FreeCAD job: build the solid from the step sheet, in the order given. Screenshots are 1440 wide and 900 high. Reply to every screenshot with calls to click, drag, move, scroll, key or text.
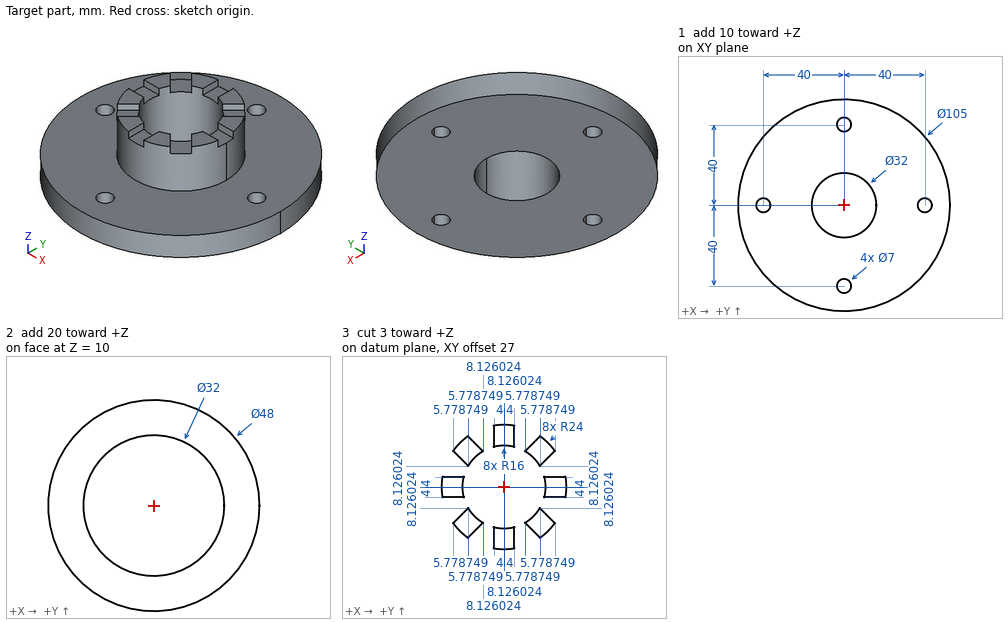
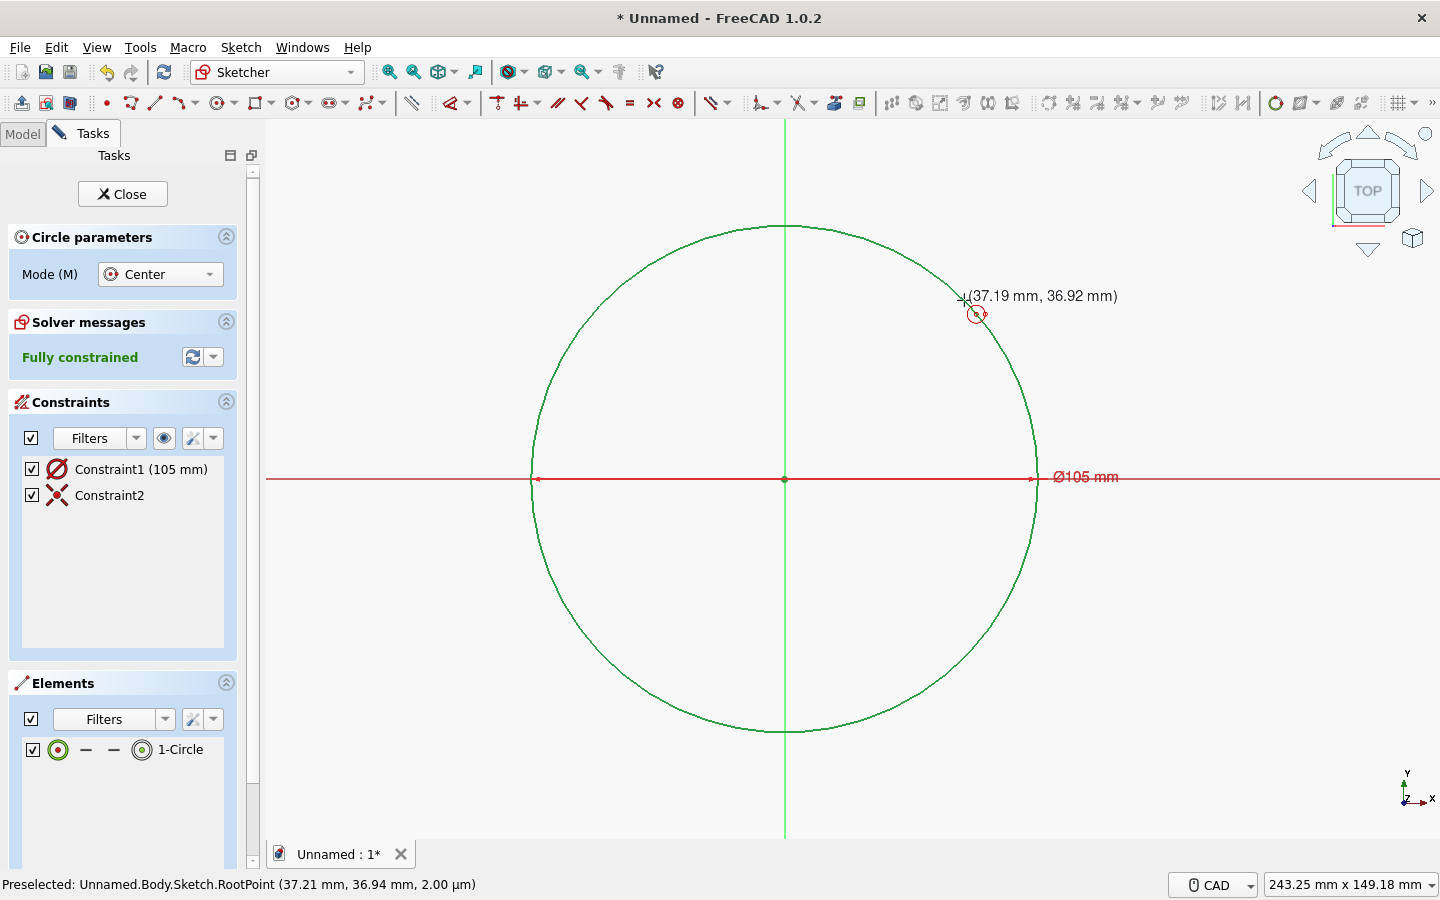
scroll(785, 672, up, 2)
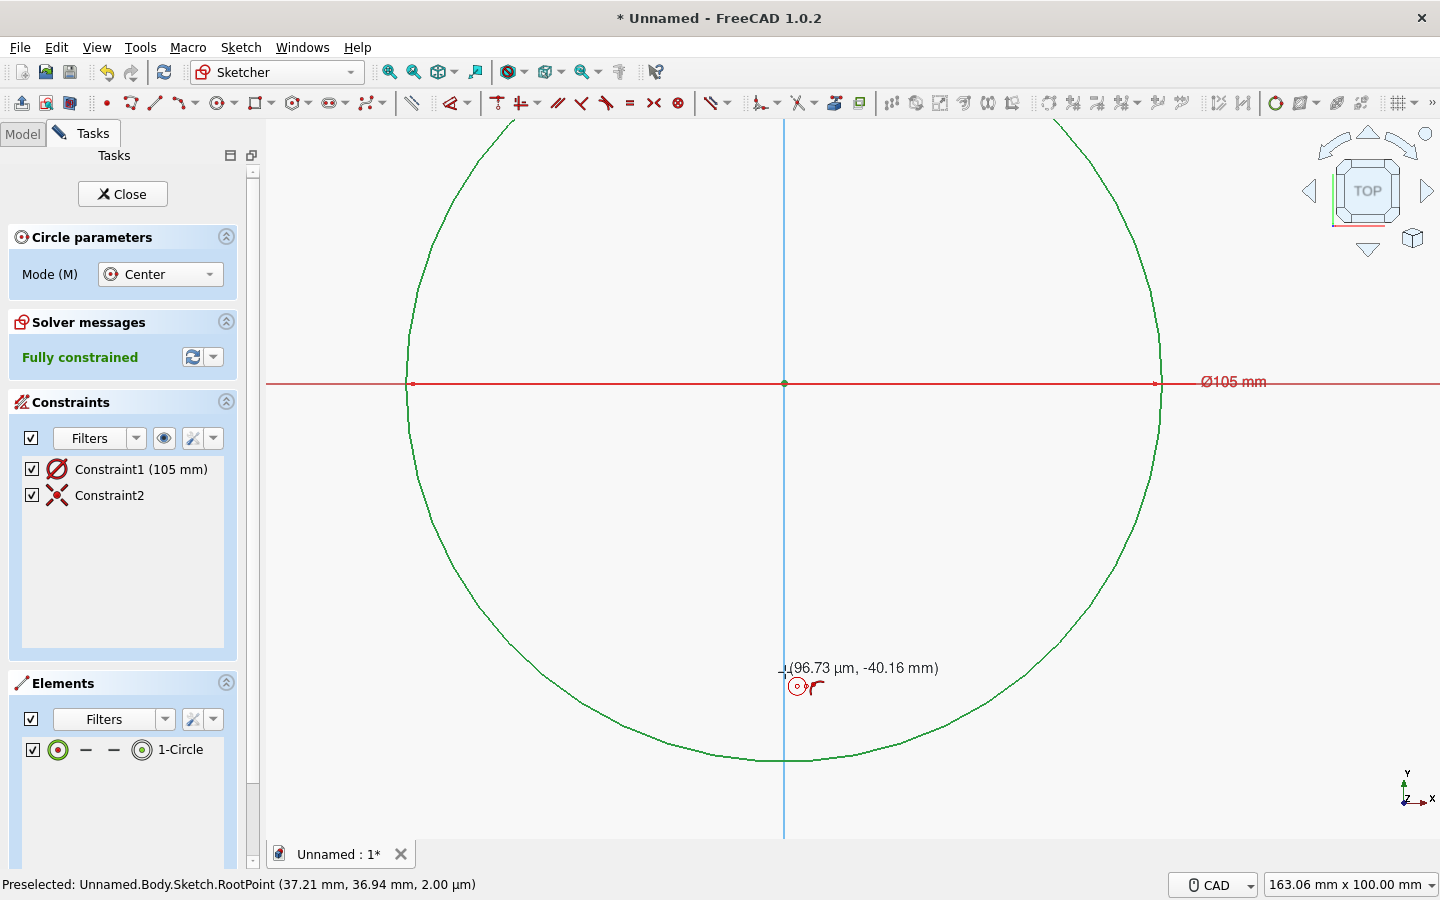
click(784, 672)
move(802, 654)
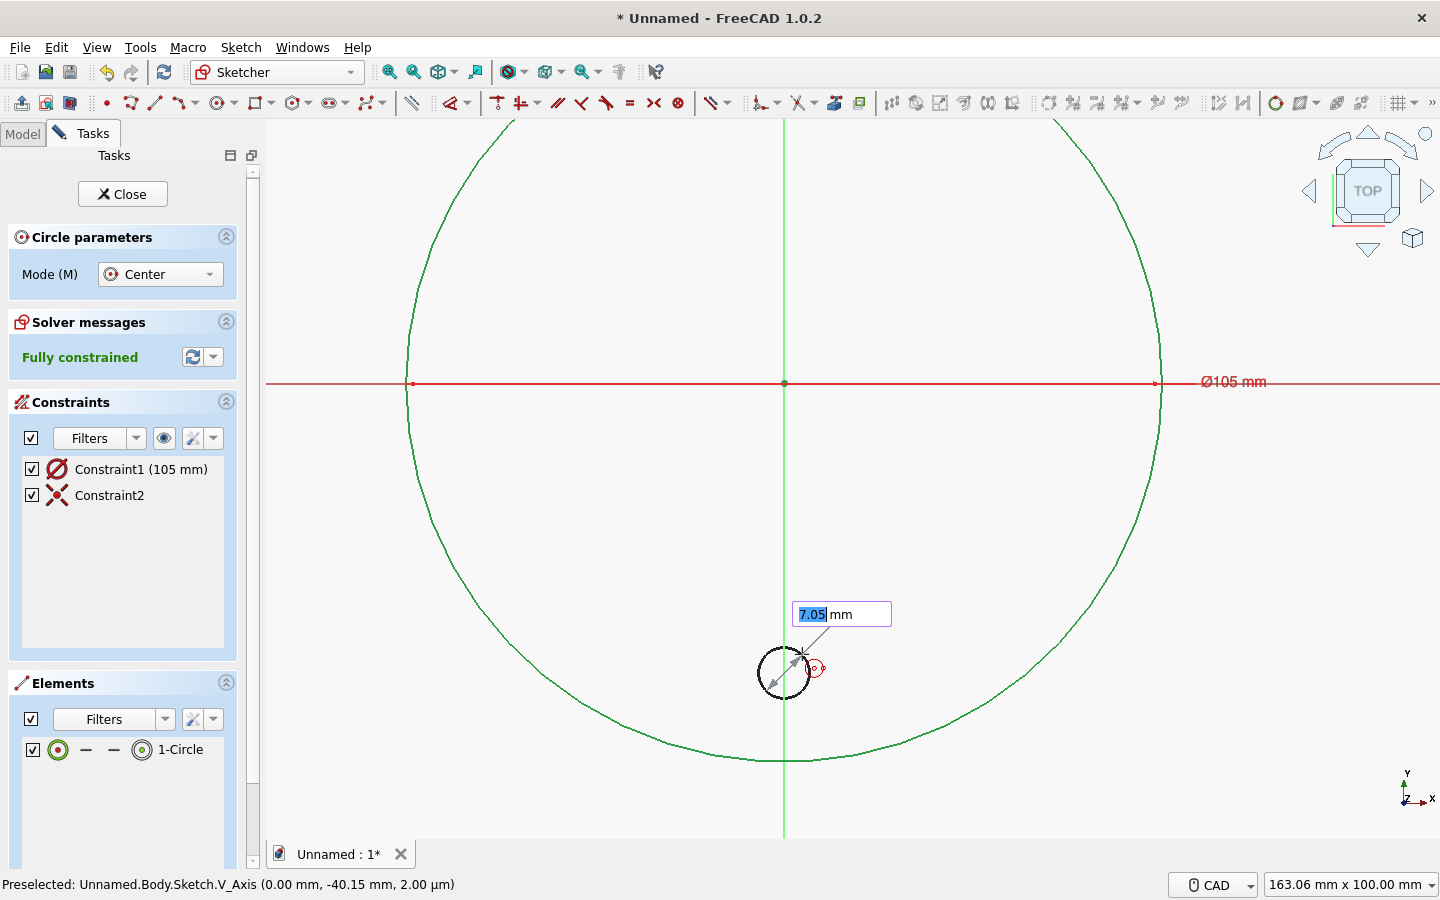
text(7)
key(Return)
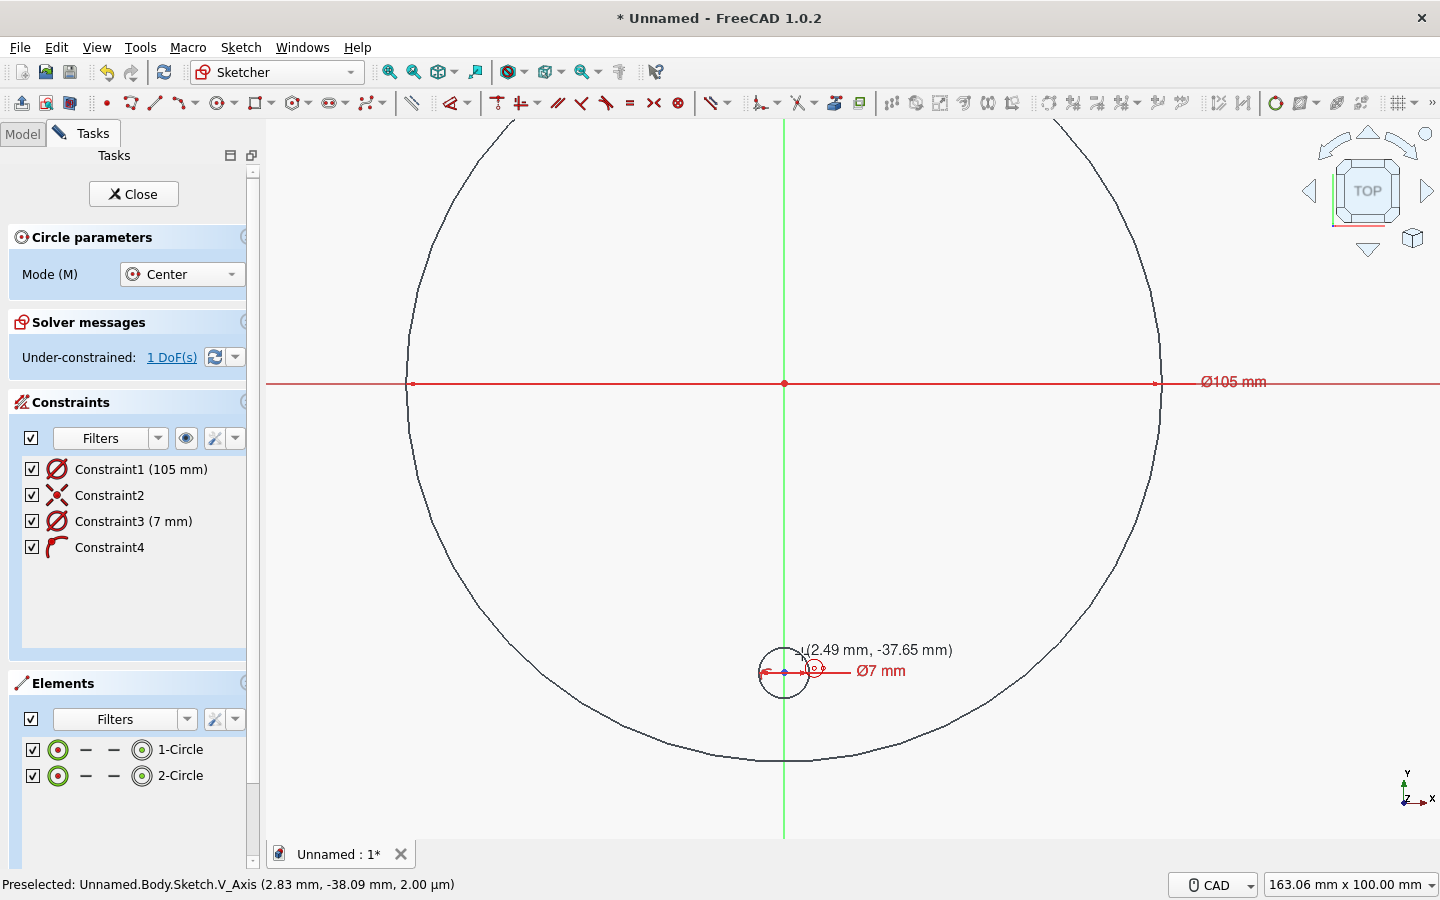
click(496, 384)
move(514, 366)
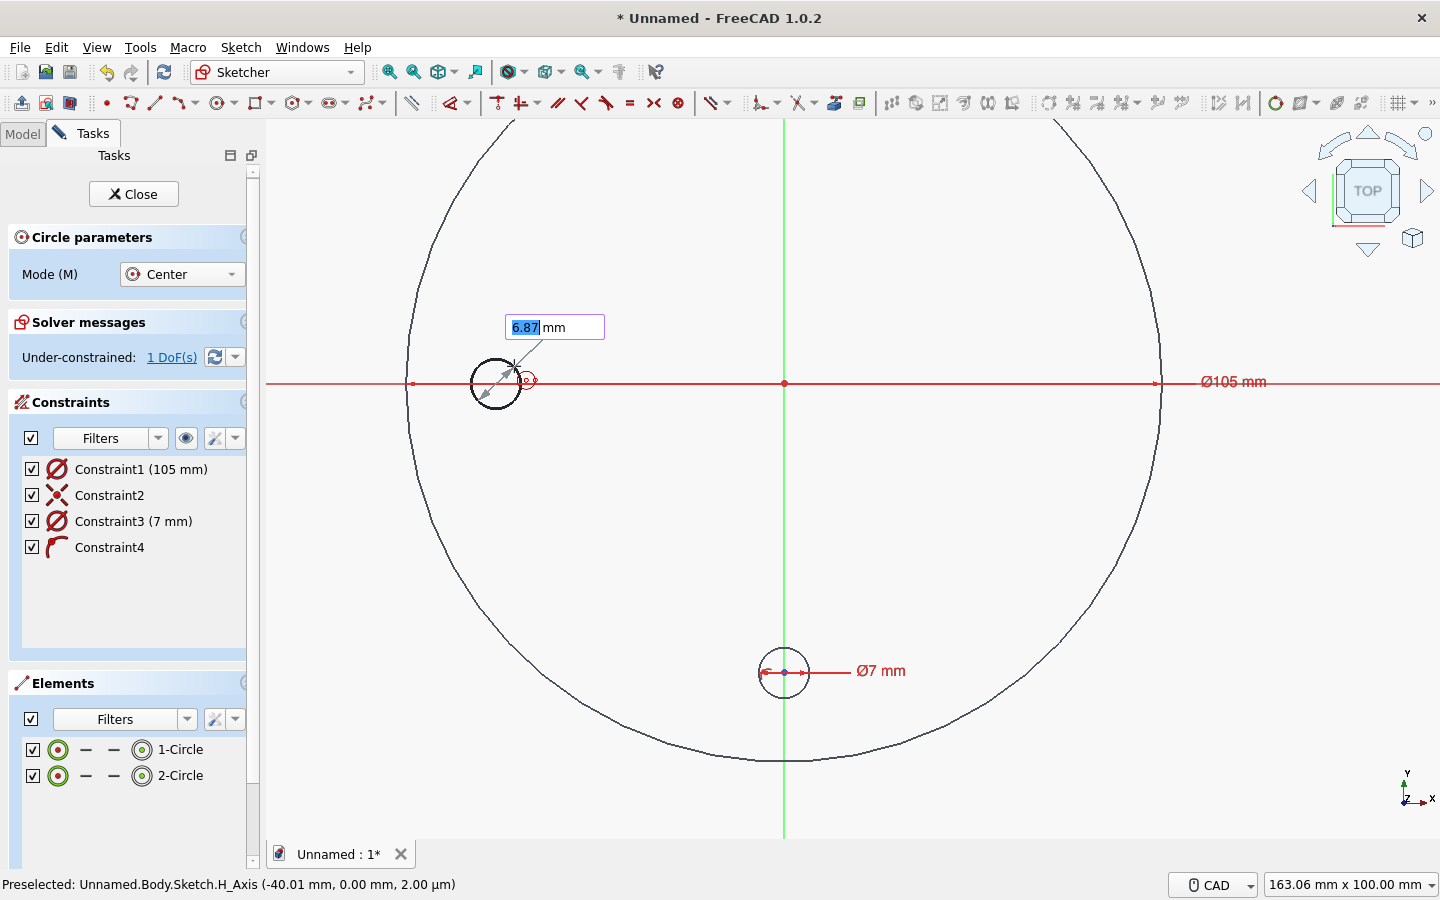
text(7)
key(Return)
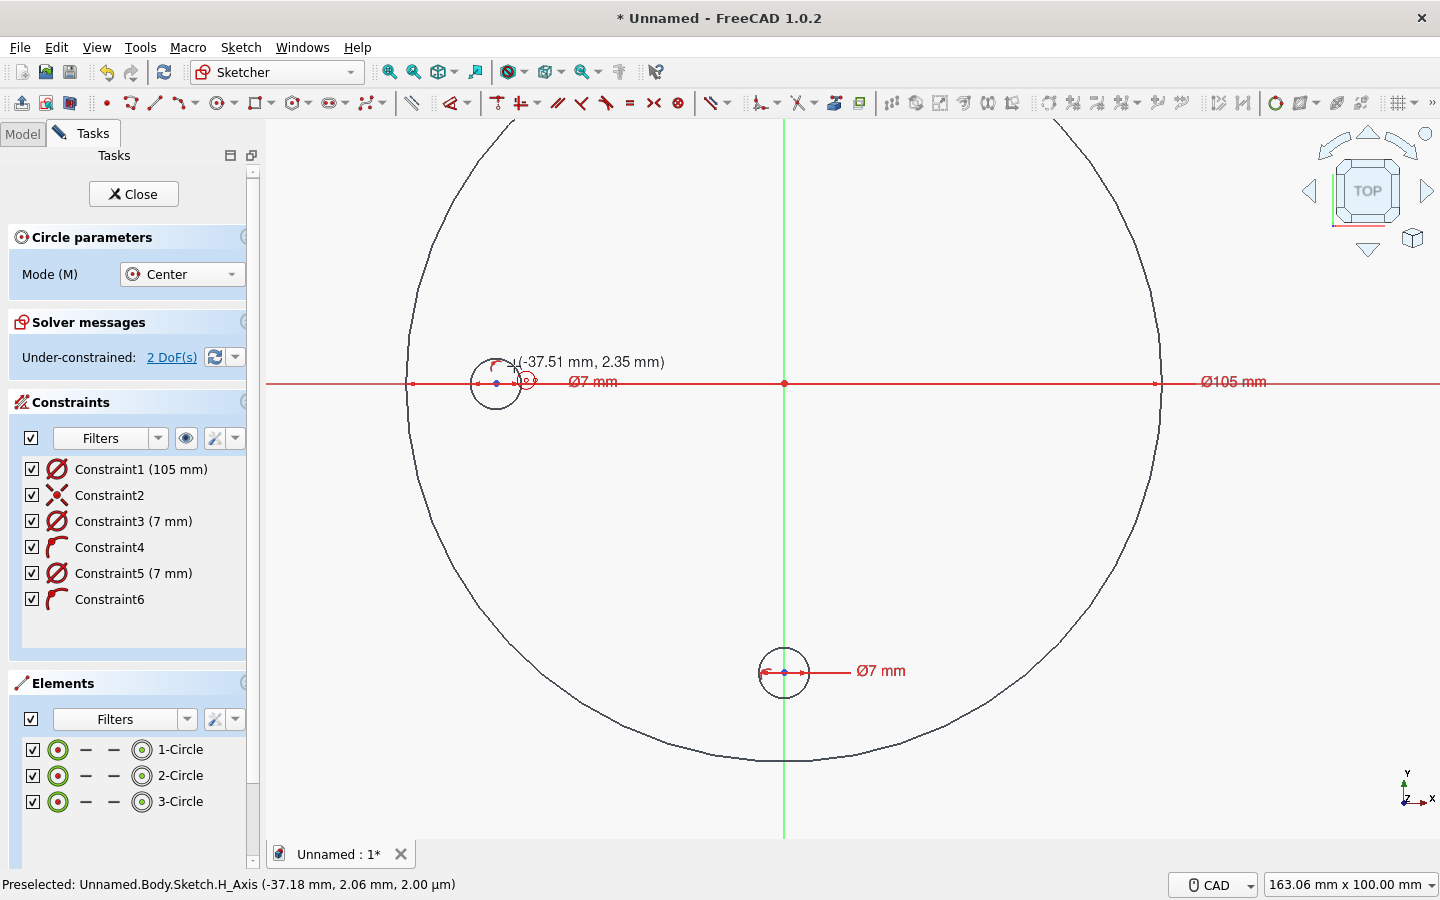
click(784, 384)
move(866, 302)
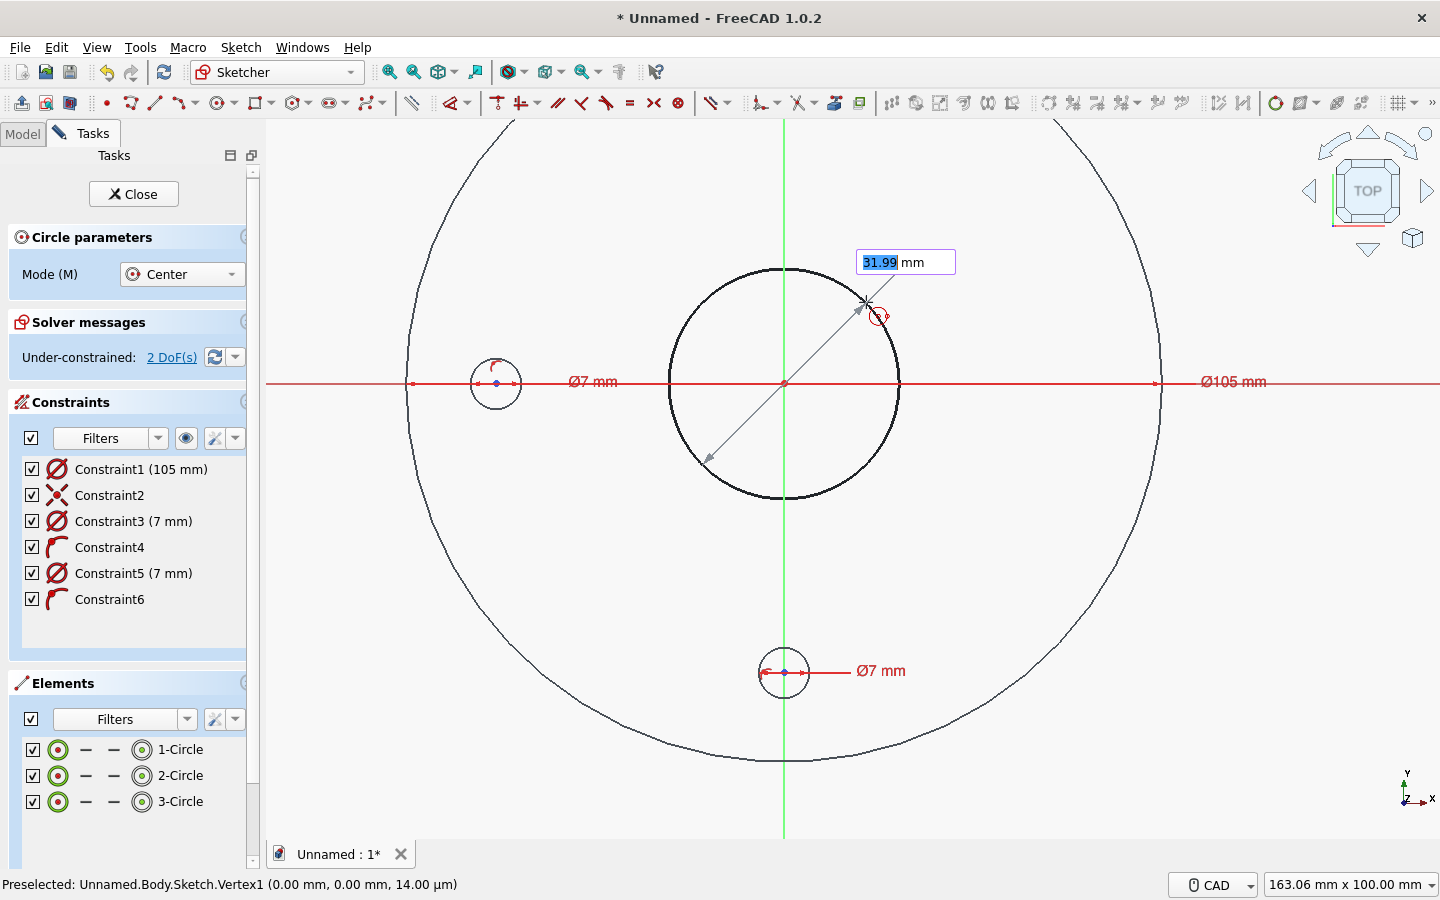
text(32)
key(Return)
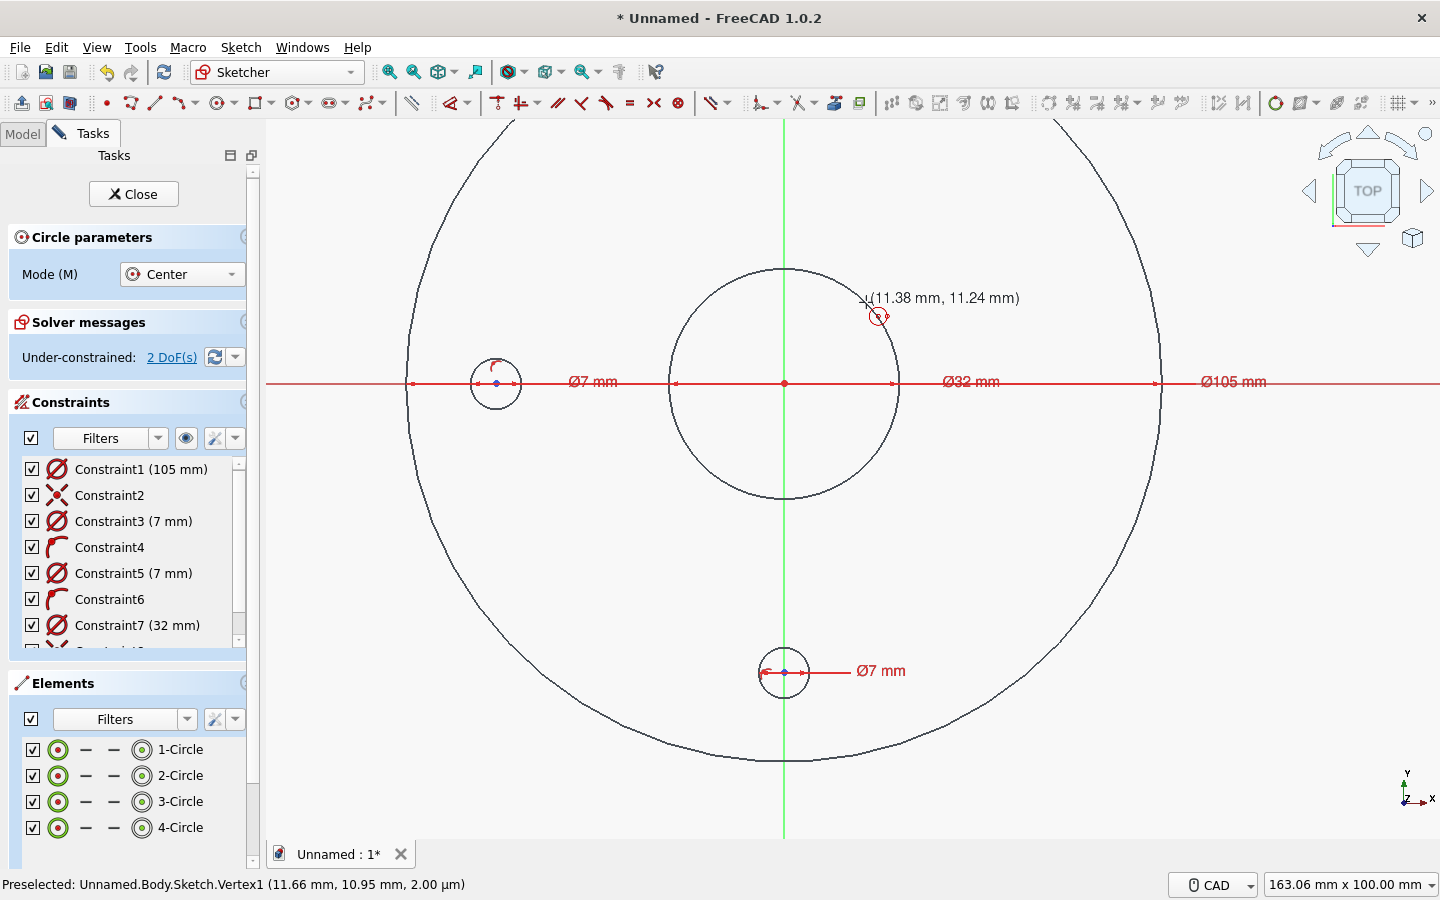
click(1072, 384)
move(1090, 366)